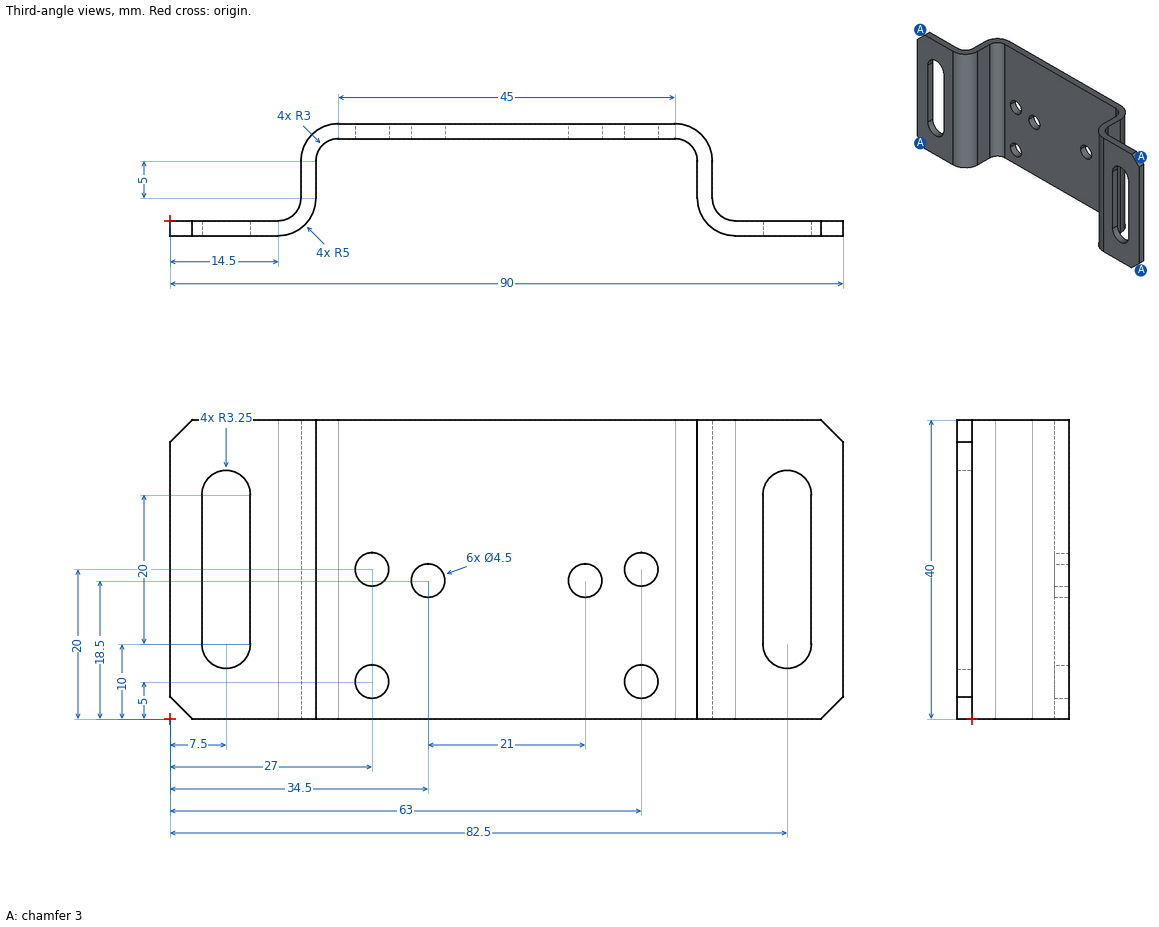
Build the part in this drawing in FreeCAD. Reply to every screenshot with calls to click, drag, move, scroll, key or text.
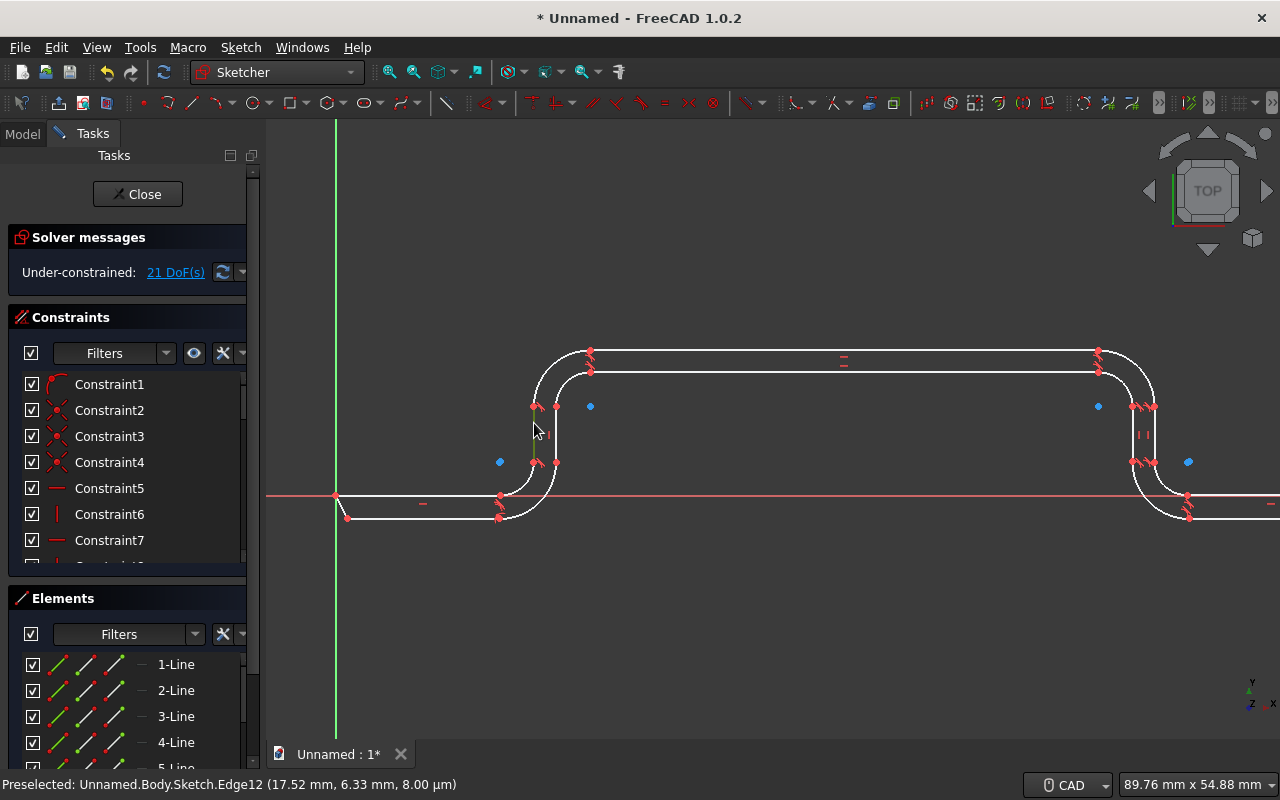
click(565, 357)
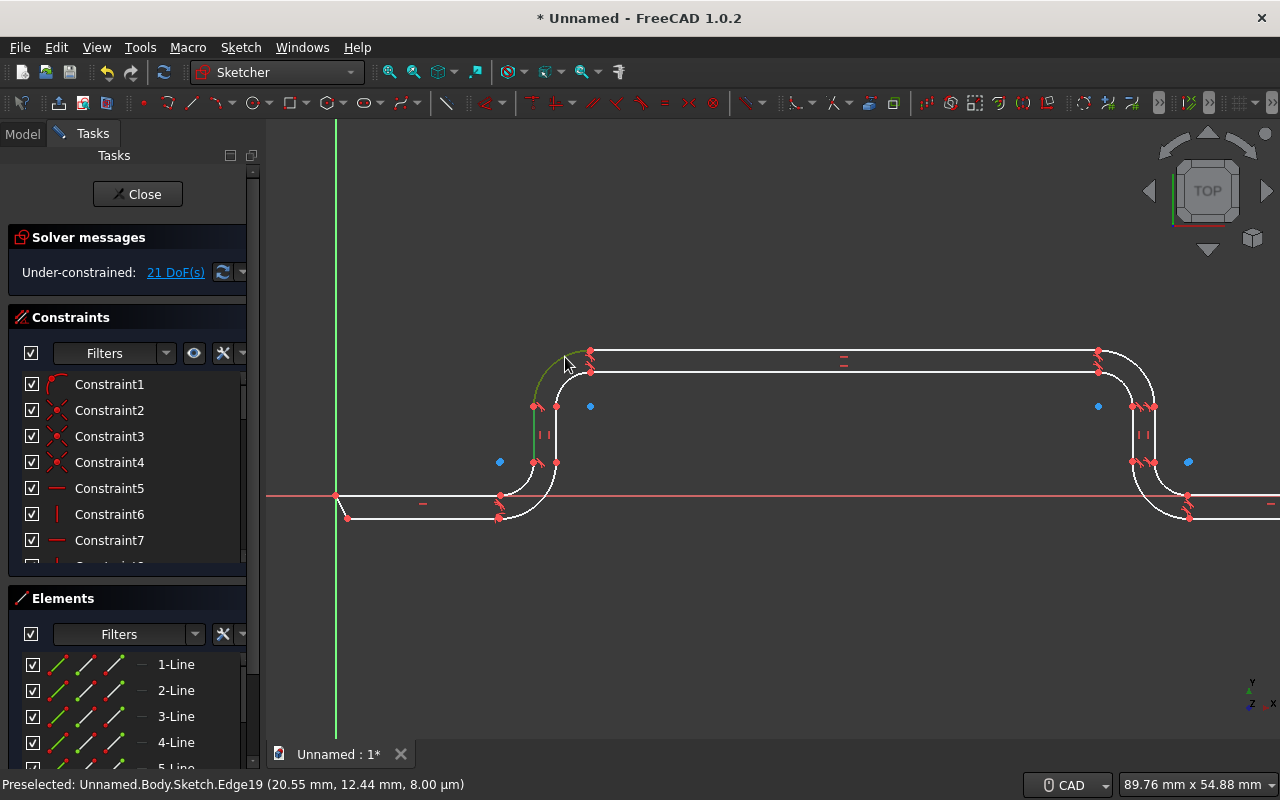
click(642, 104)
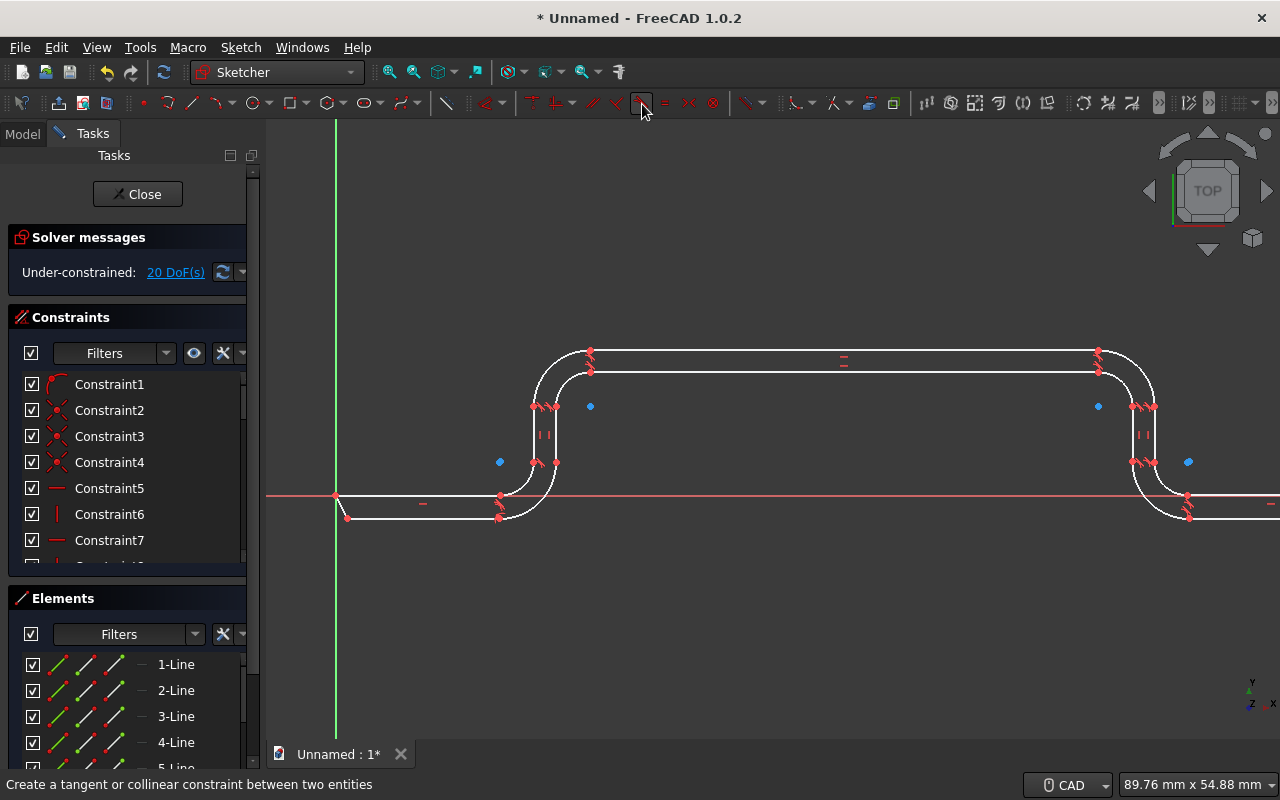
click(534, 424)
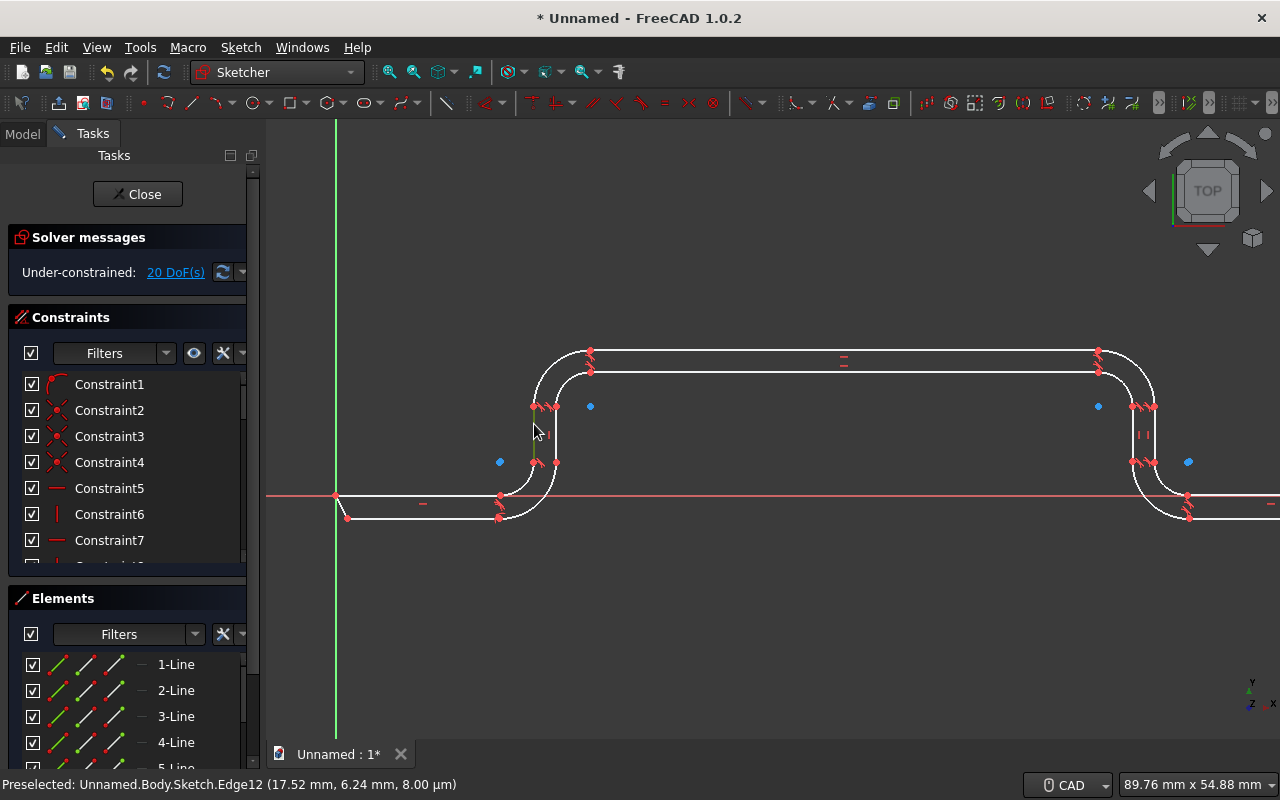
click(515, 492)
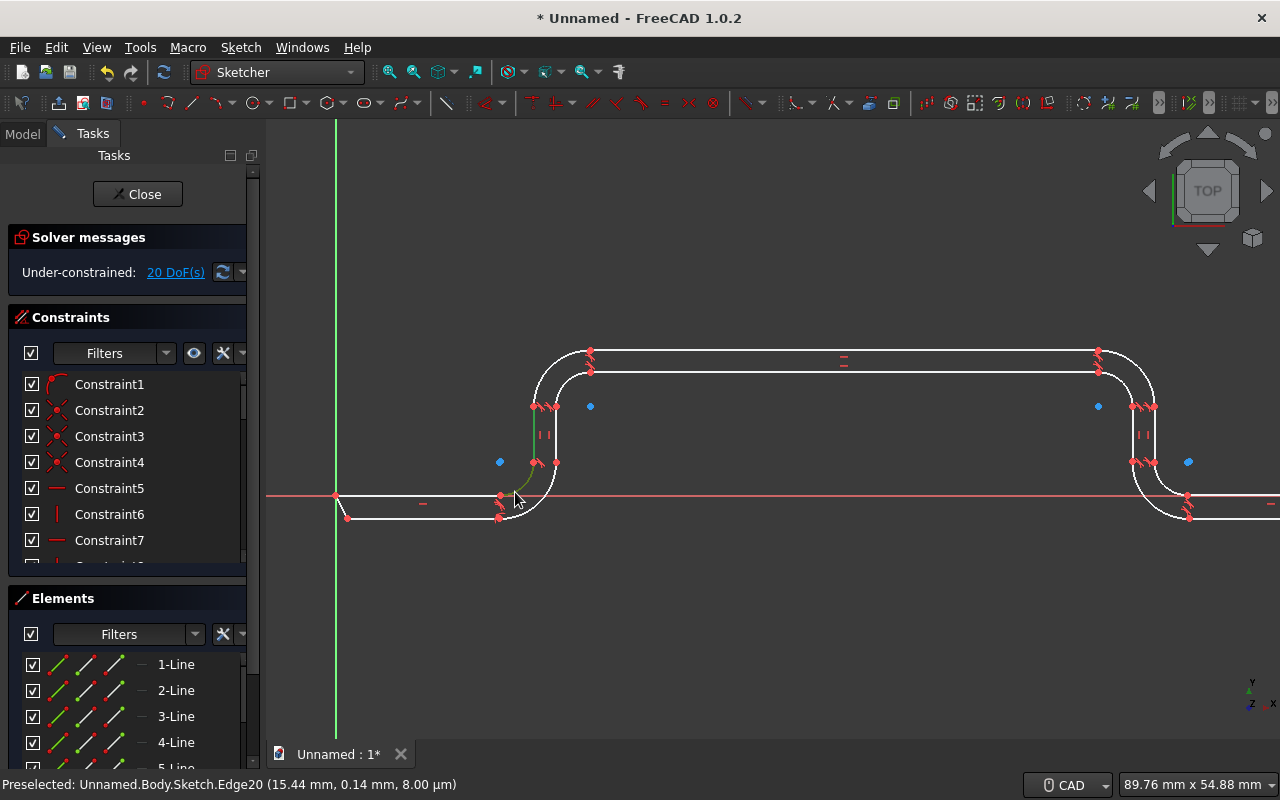
key(t)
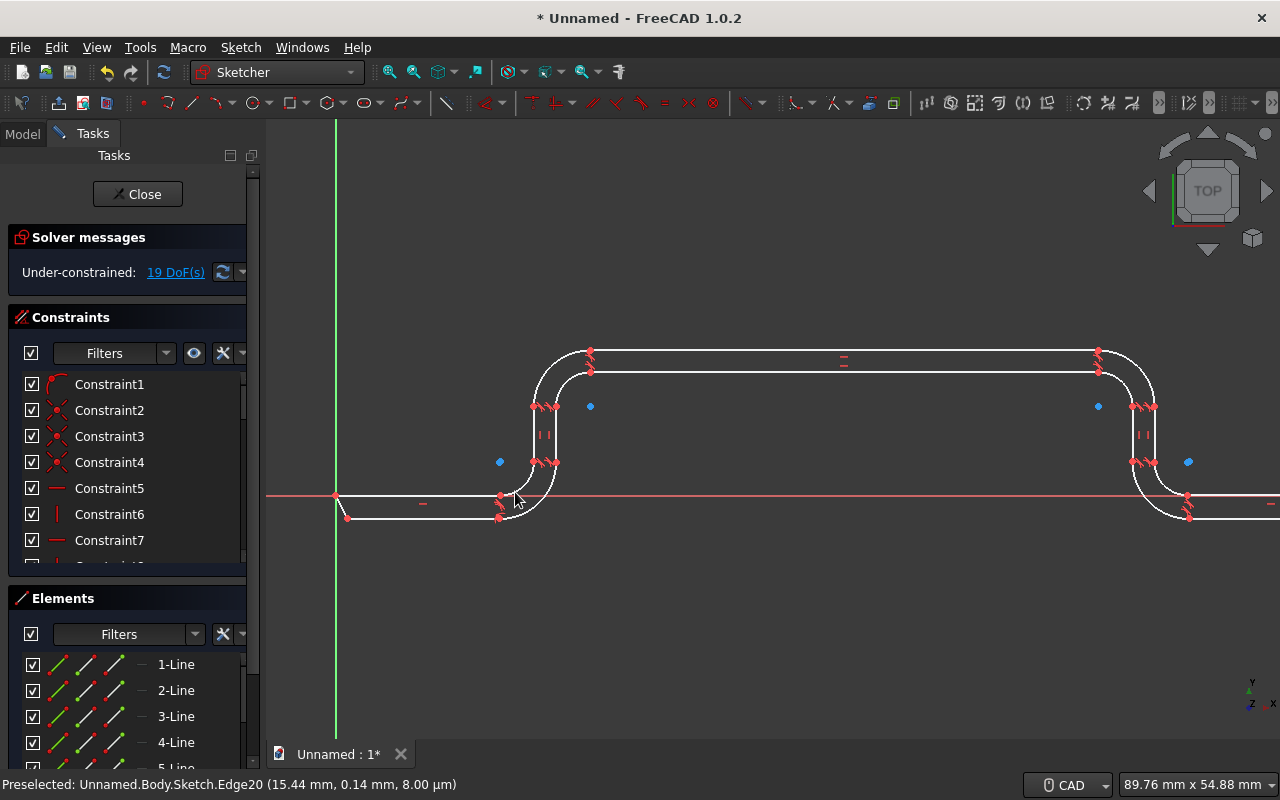
scroll(344, 512, up, 3)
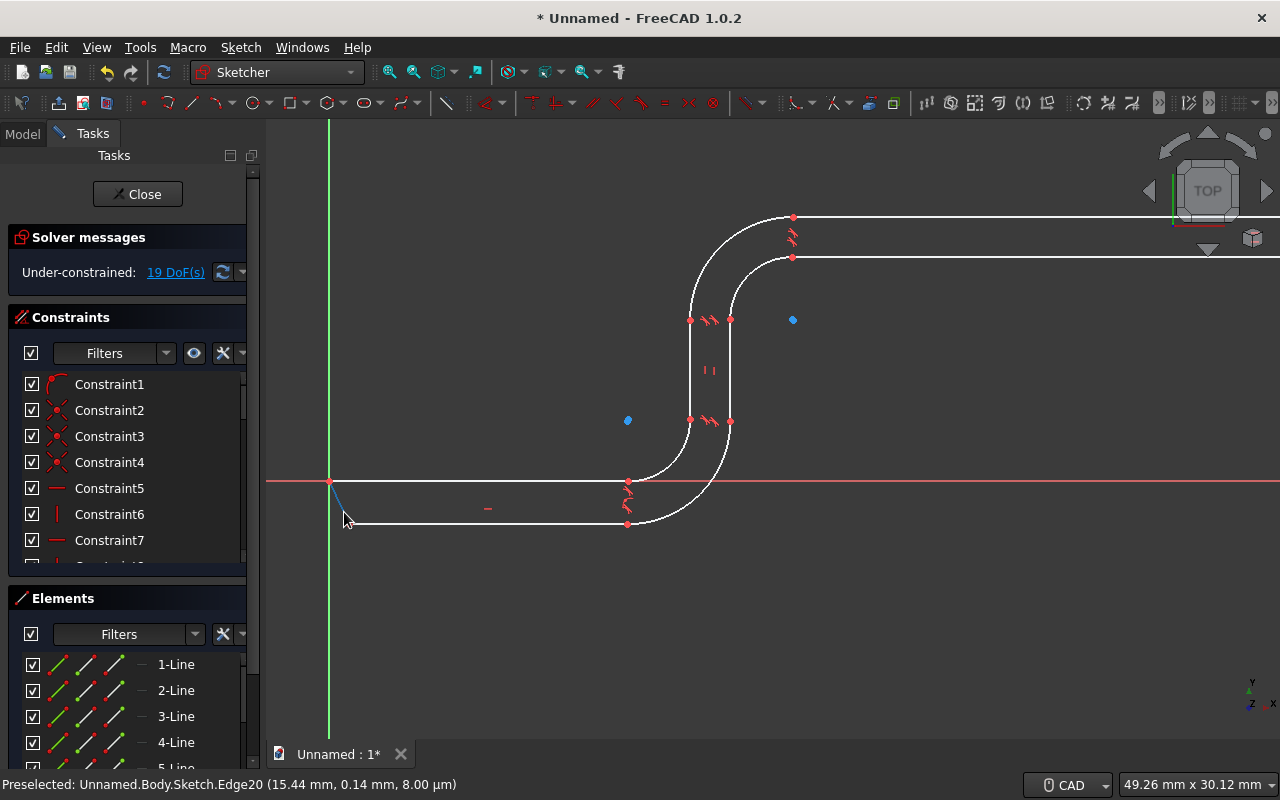
click(344, 511)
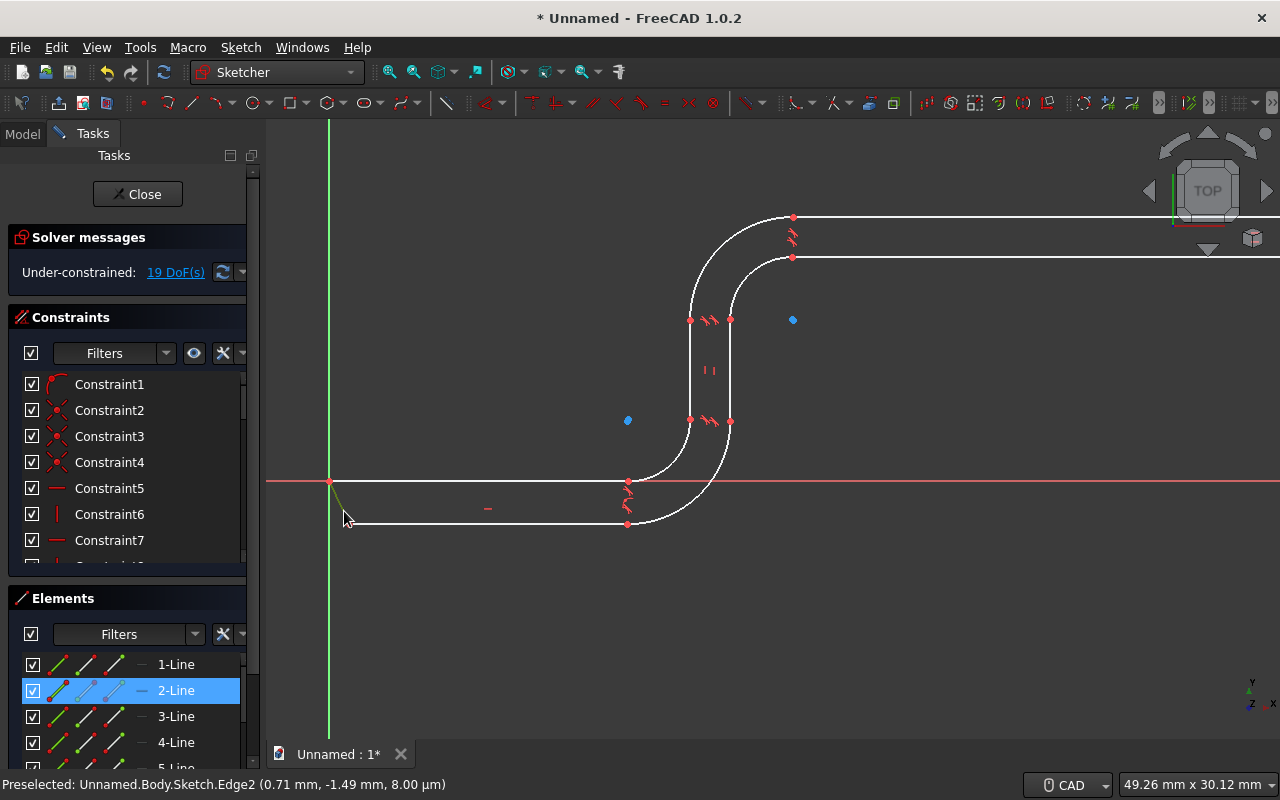
key(v)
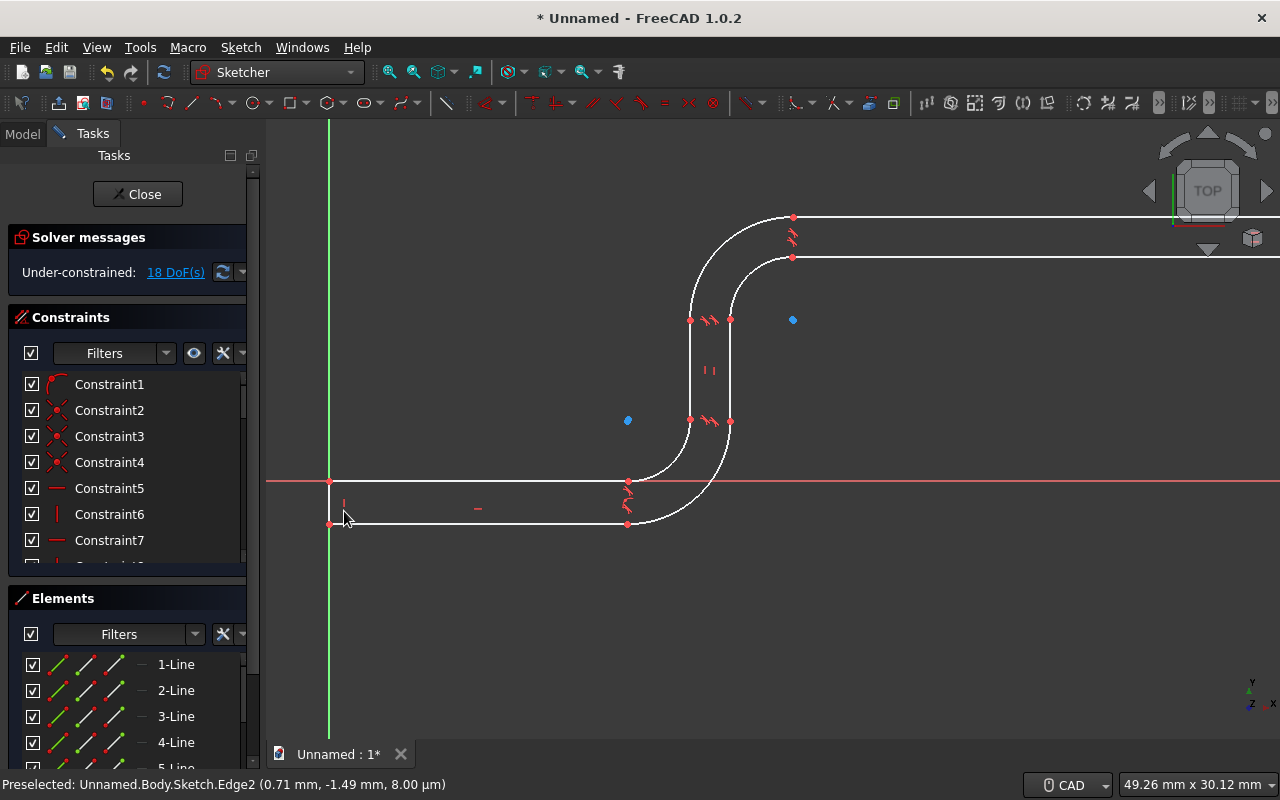
scroll(467, 455, down, 6)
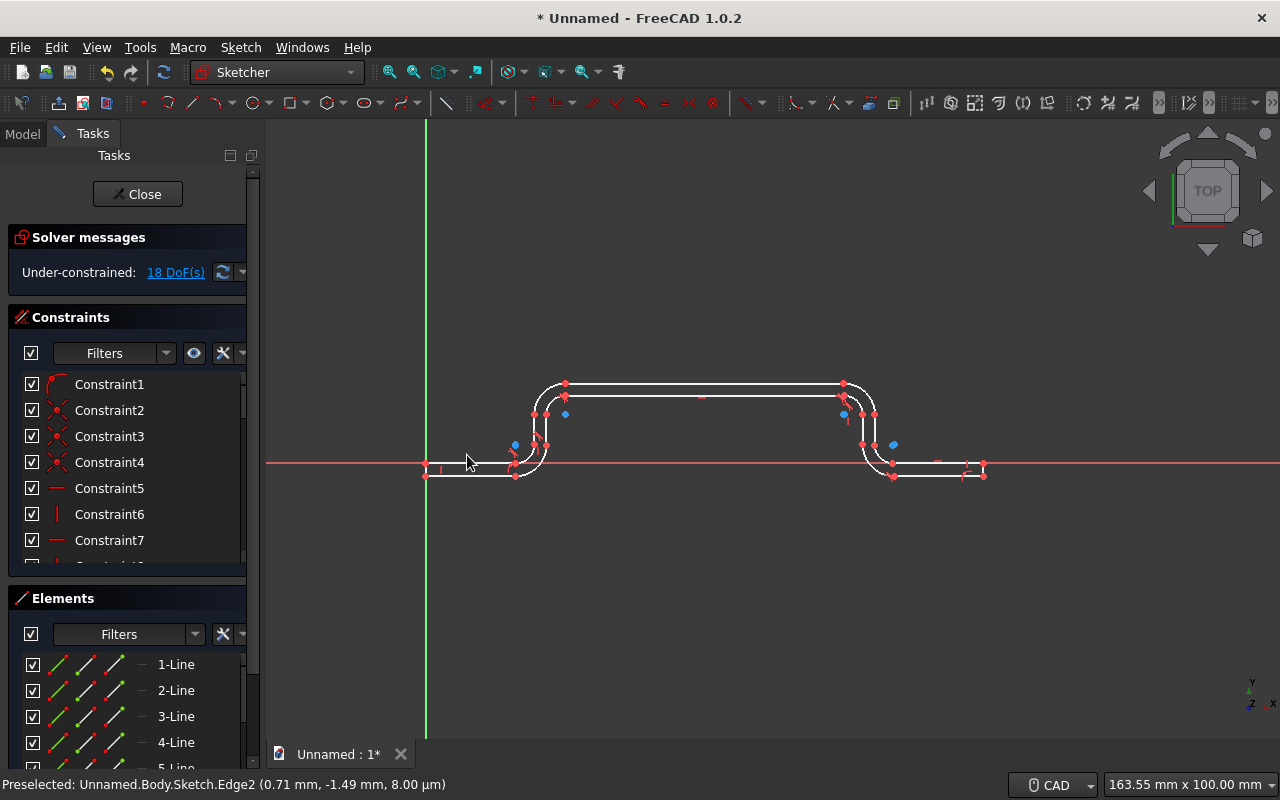
click(956, 463)